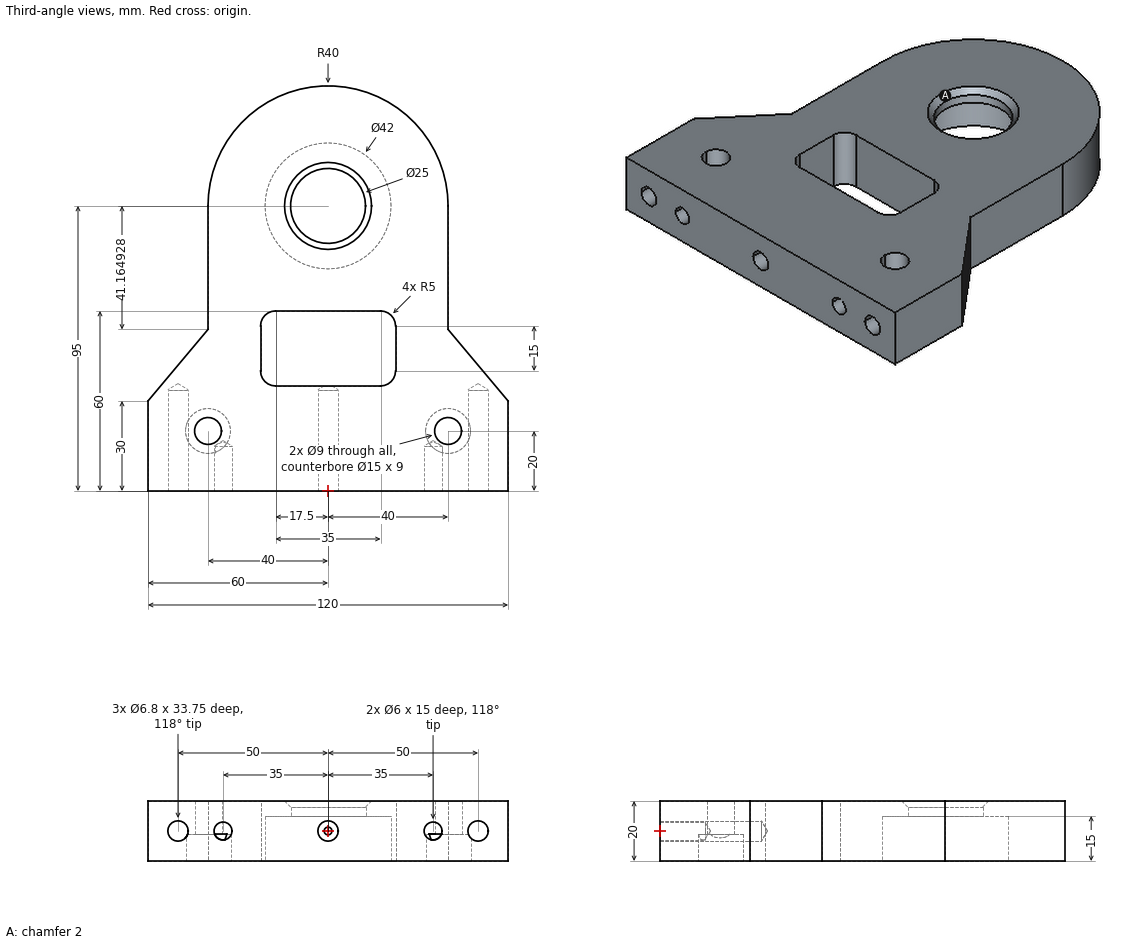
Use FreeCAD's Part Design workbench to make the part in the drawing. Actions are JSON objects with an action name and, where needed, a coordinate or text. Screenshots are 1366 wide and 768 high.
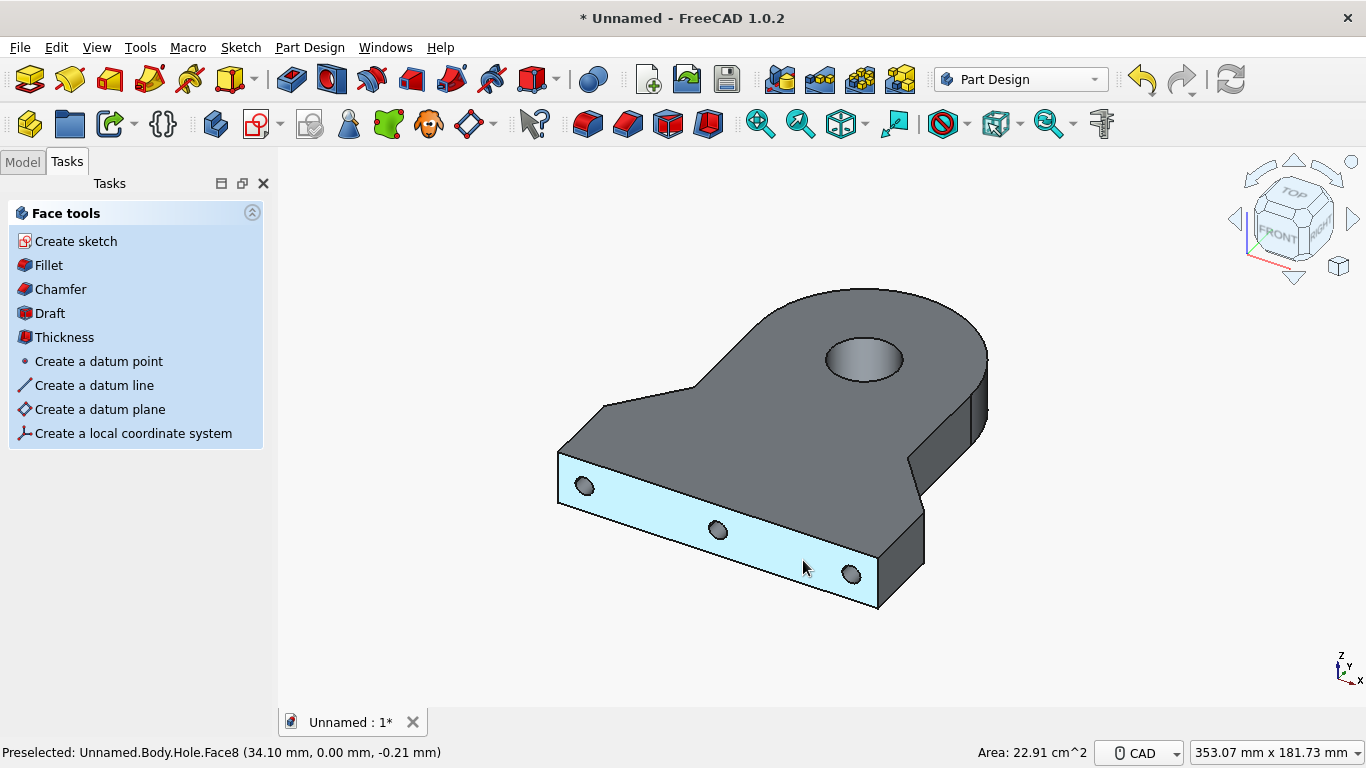
{"action": "left_click", "coordinate": [256, 124]}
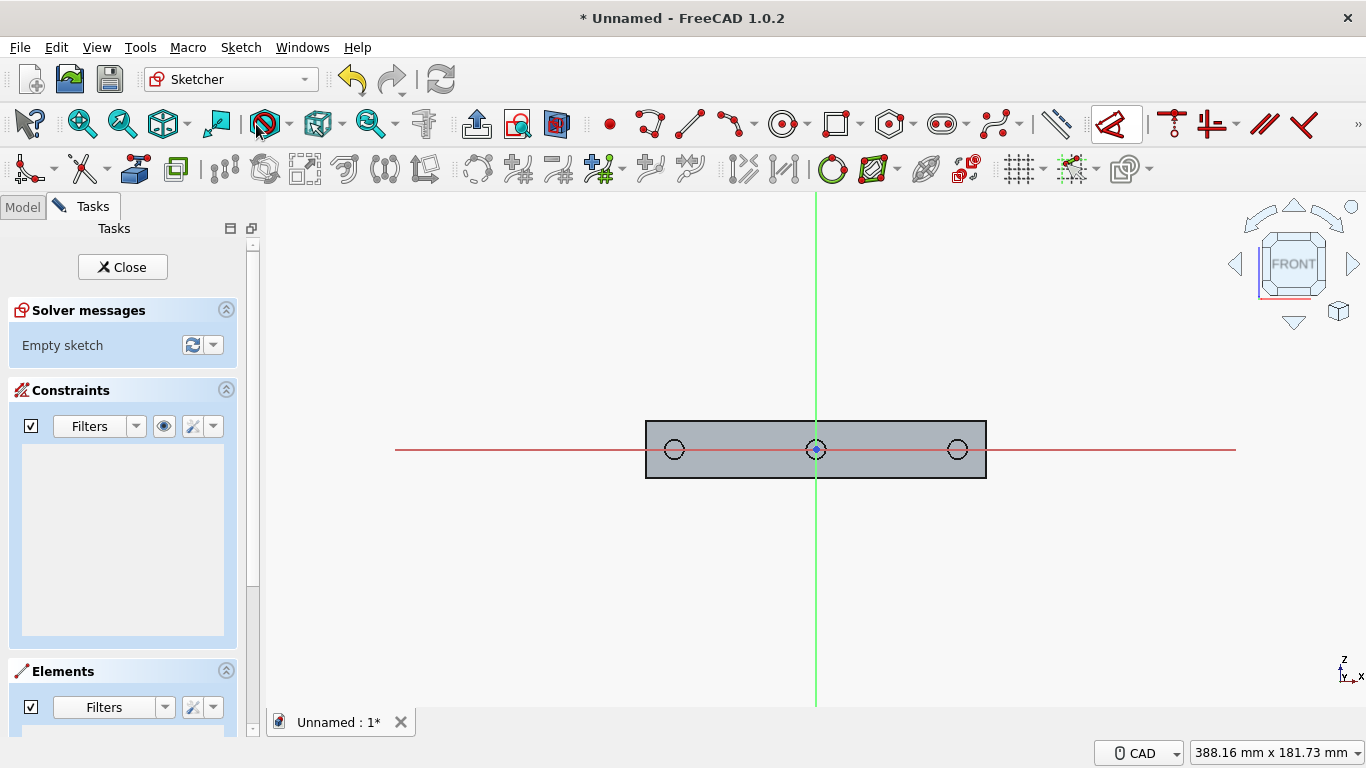
{"action": "scroll", "coordinate": [856, 450], "scroll_direction": "up", "scroll_amount": 5}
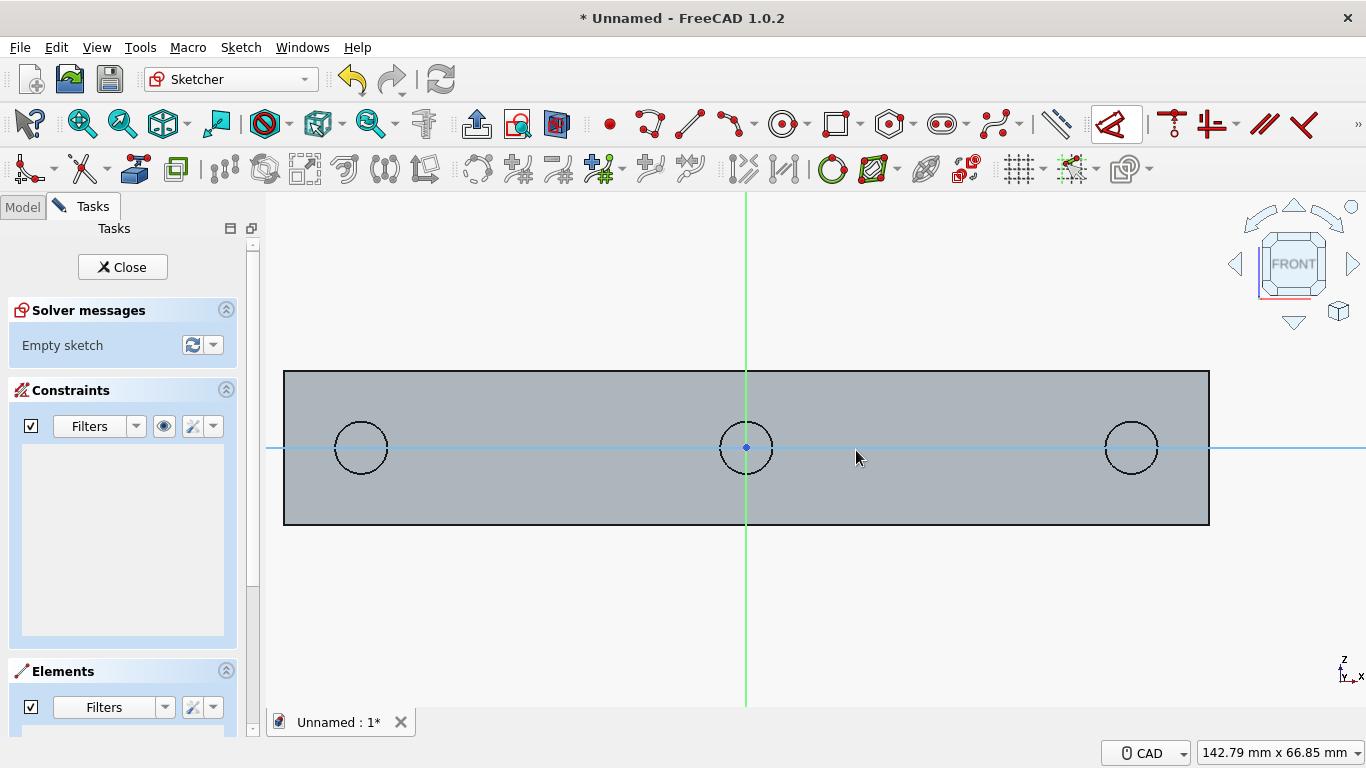
{"action": "key", "text": "g c"}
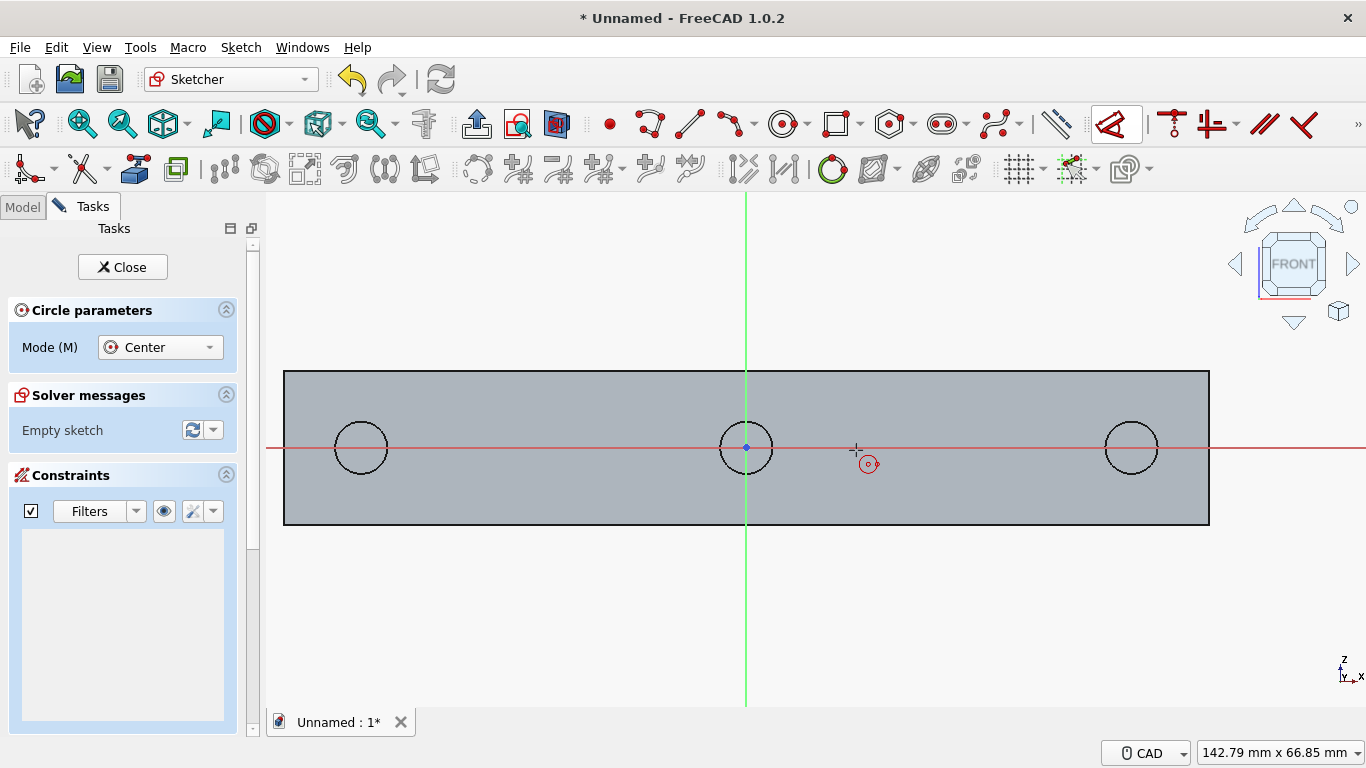
{"action": "left_click", "coordinate": [1016, 448]}
{"action": "left_click", "coordinate": [1032, 431]}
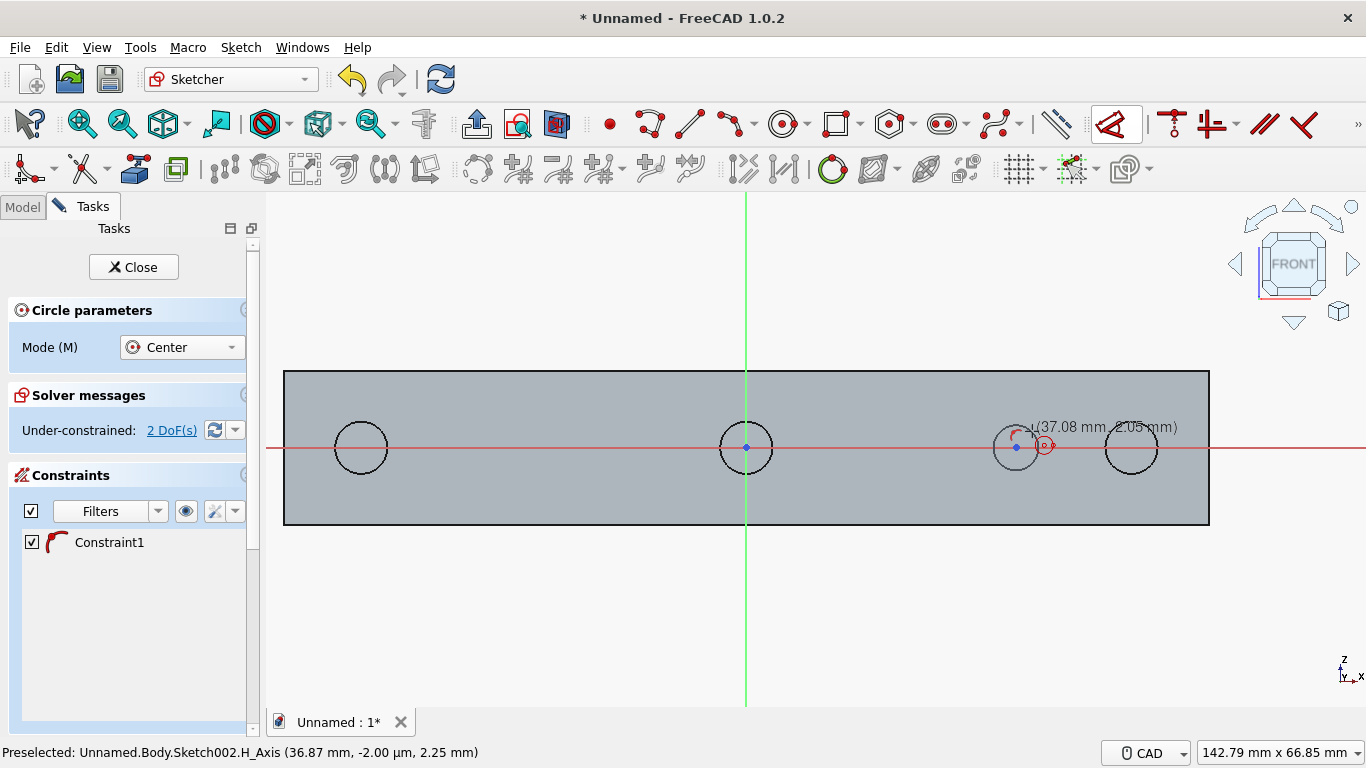
{"action": "left_click", "coordinate": [477, 448]}
{"action": "left_click", "coordinate": [493, 431]}
{"action": "key", "text": "Escape"}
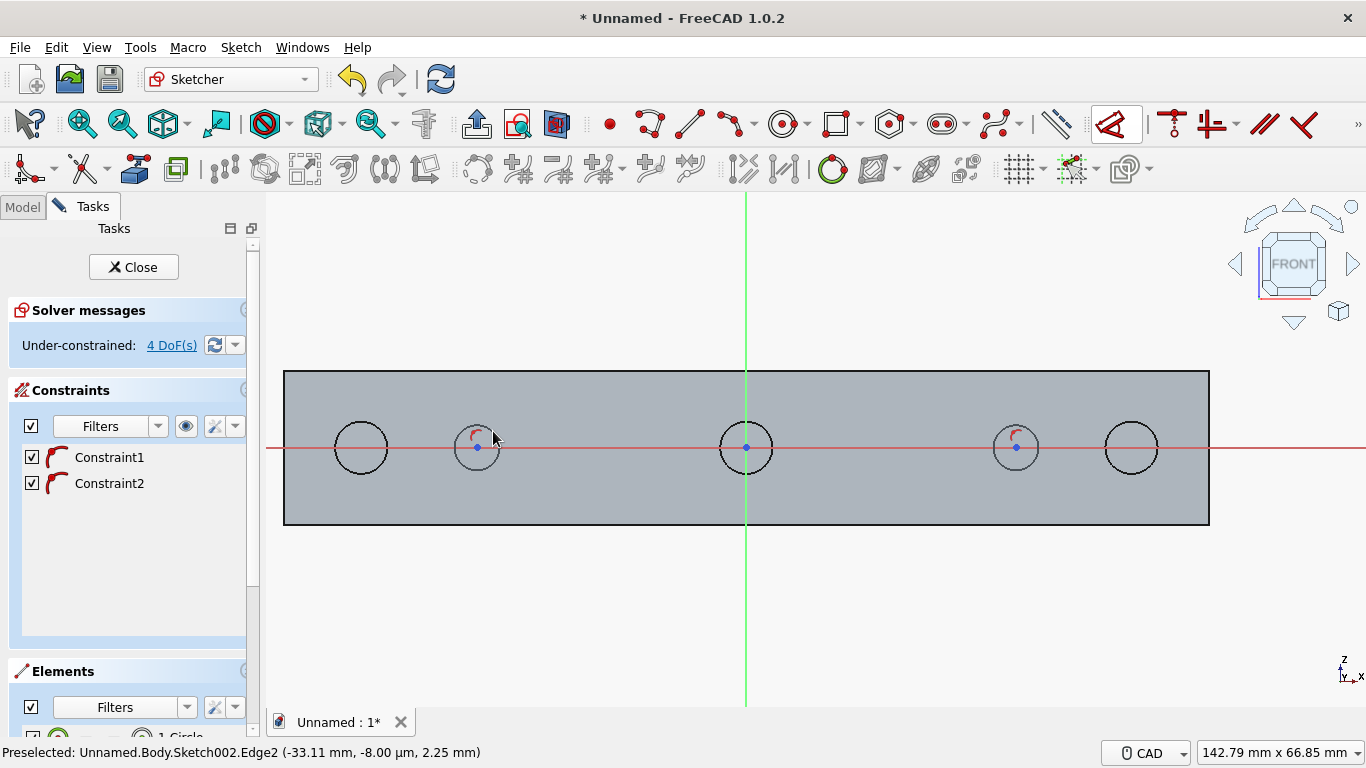
{"action": "left_click", "coordinate": [1032, 432]}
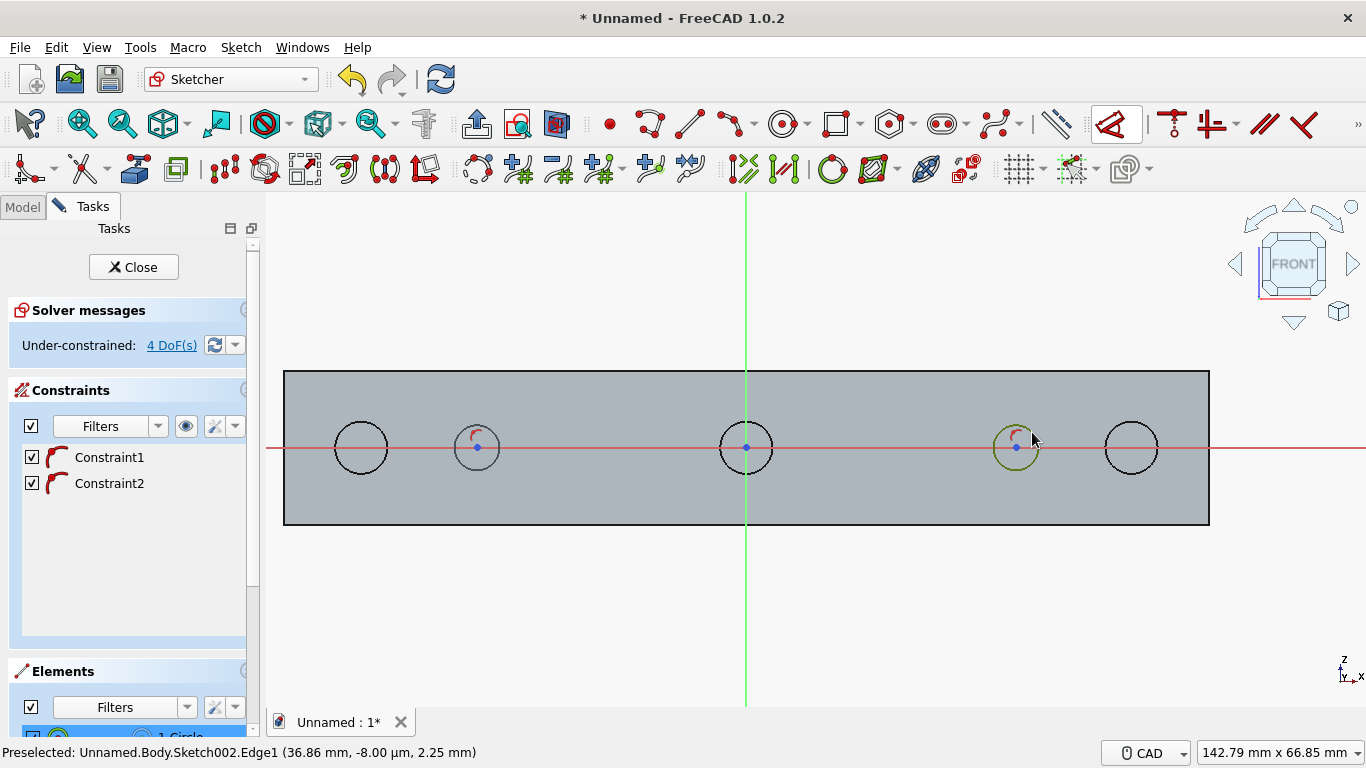
{"action": "left_click", "coordinate": [493, 432]}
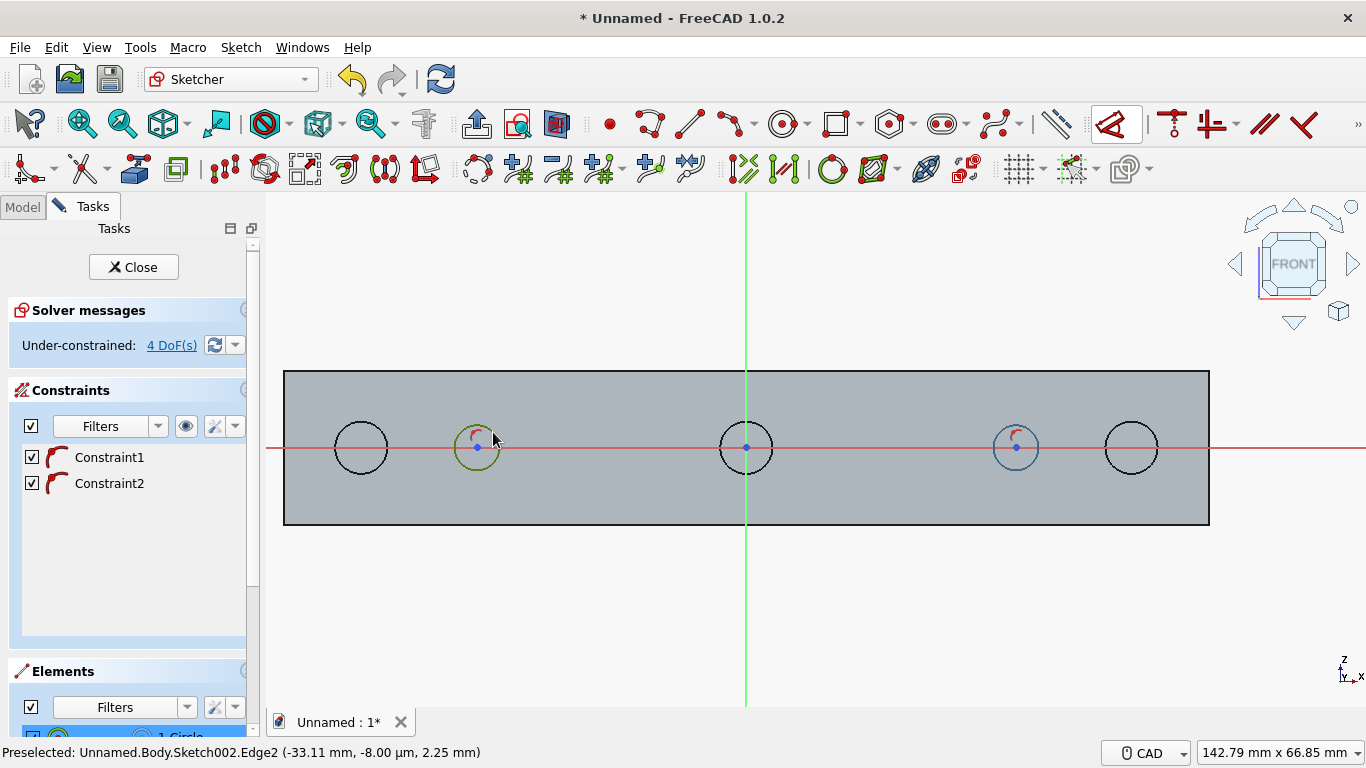
{"action": "key", "text": "e"}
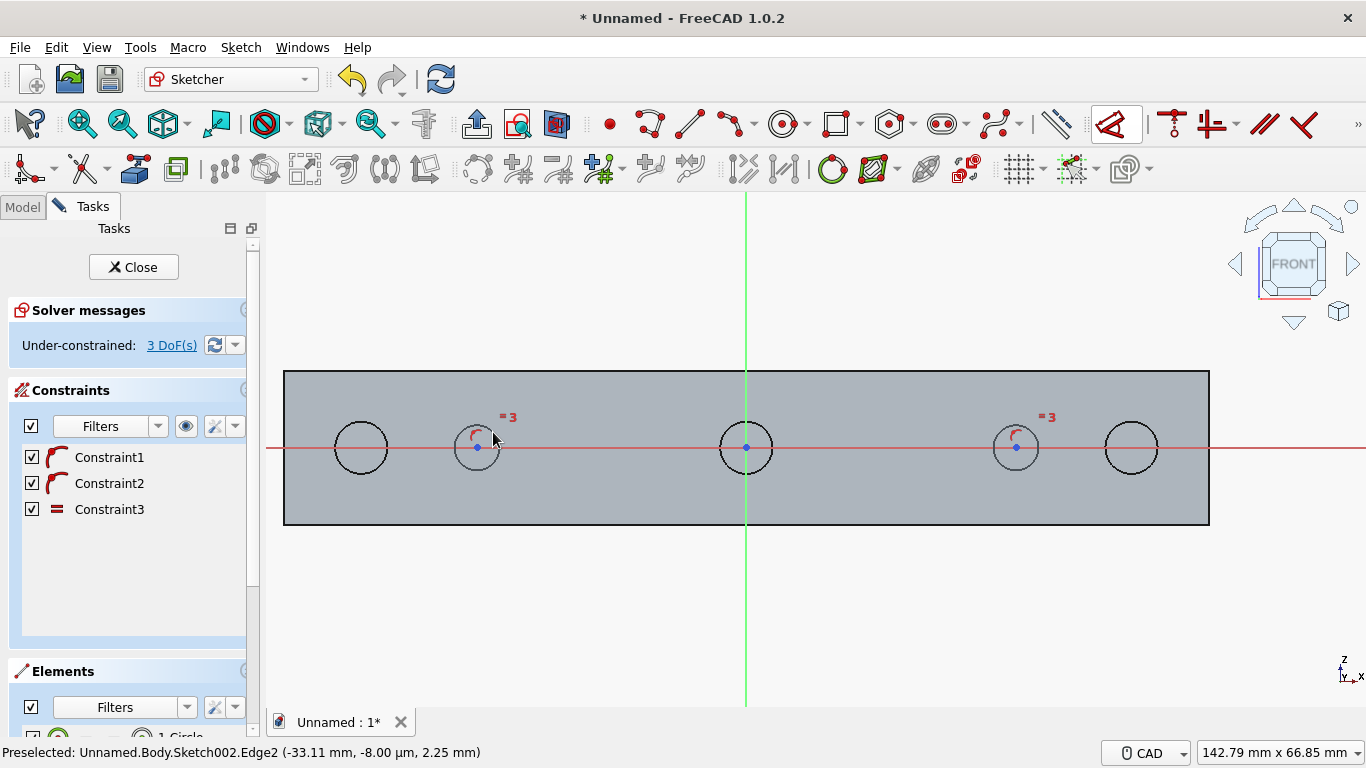
{"action": "left_click", "coordinate": [1032, 432]}